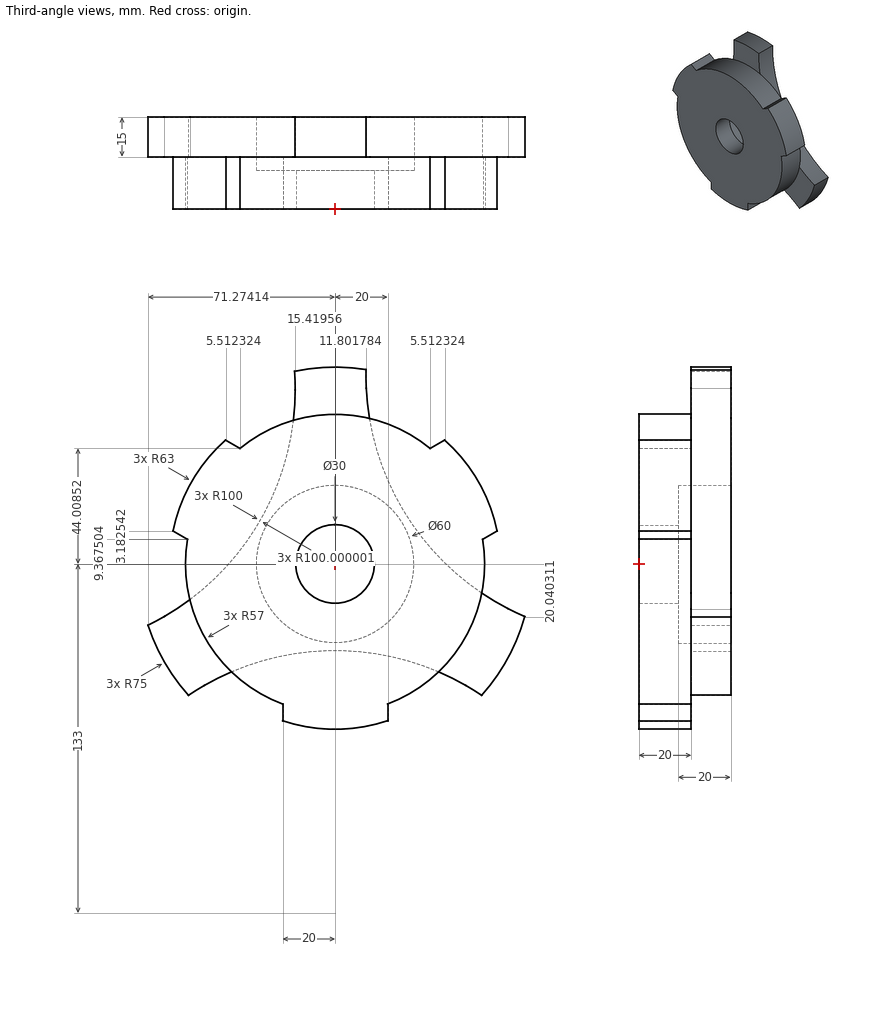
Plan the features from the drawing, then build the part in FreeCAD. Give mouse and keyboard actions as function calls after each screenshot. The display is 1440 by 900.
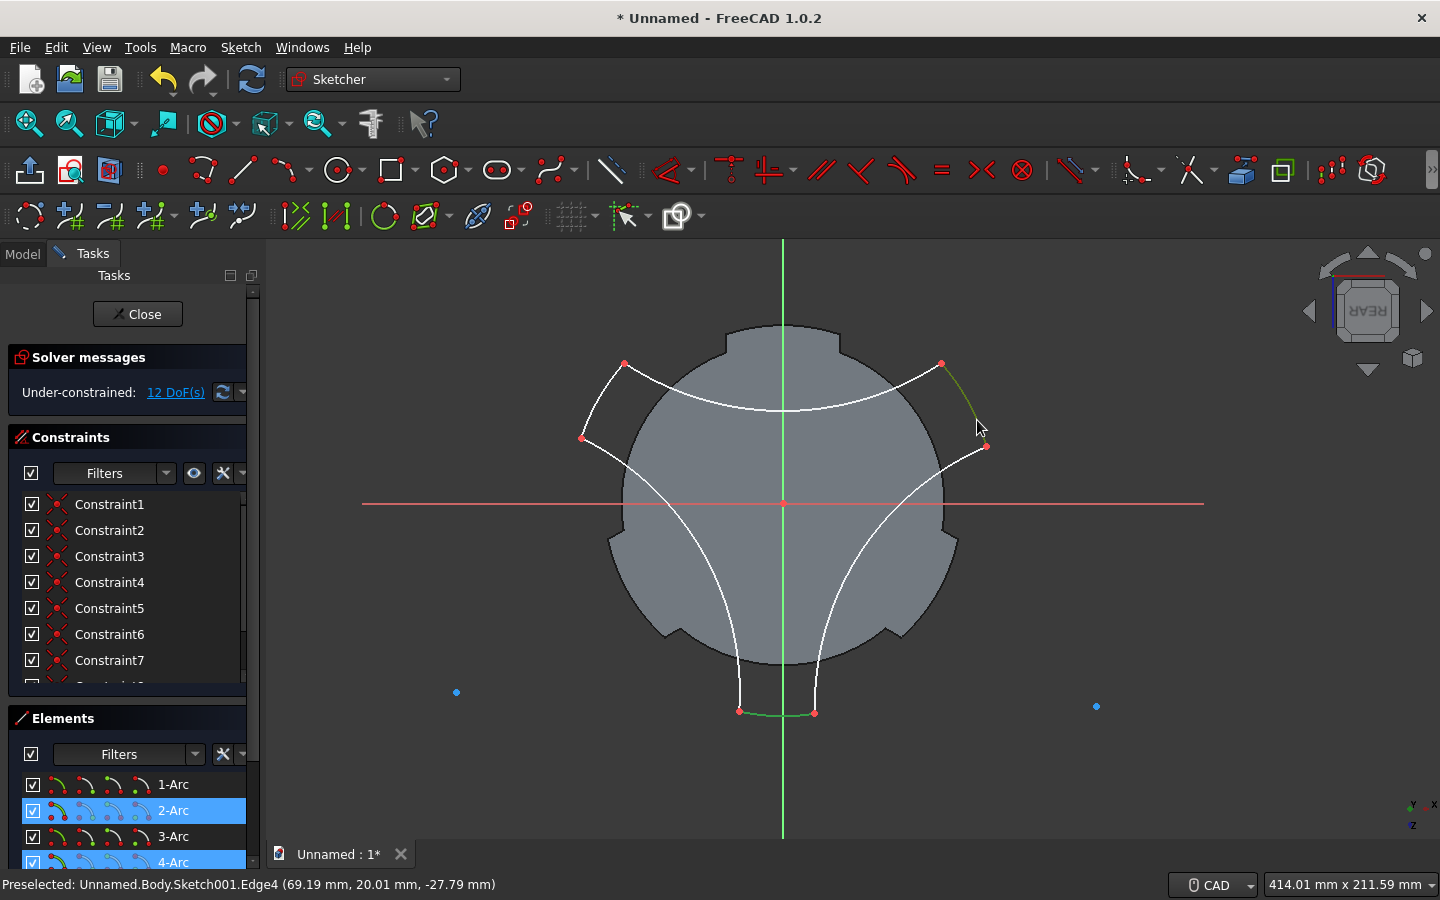
click(608, 384)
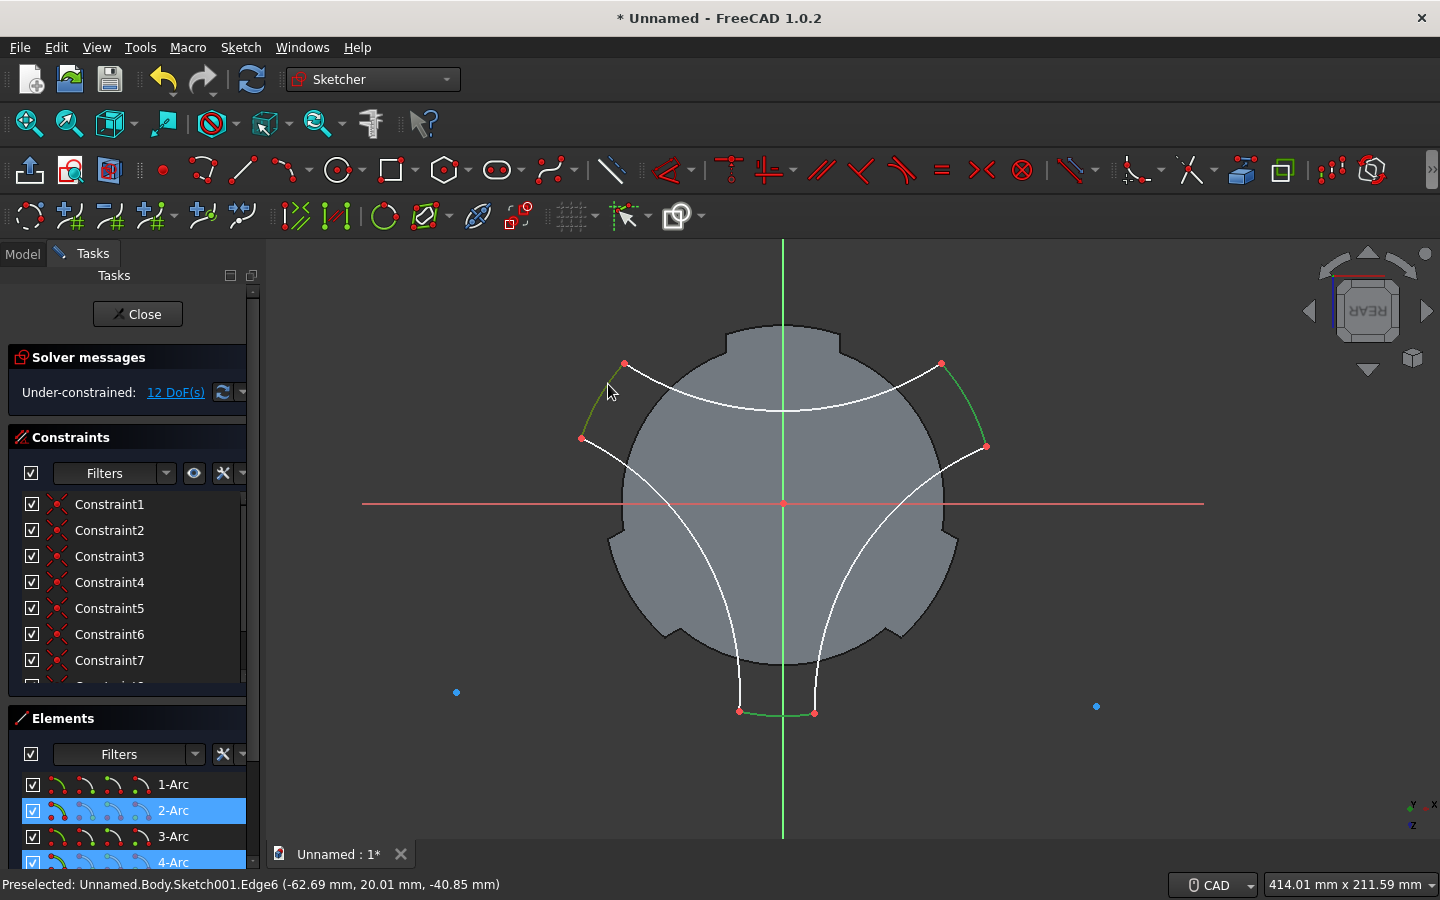
click(942, 170)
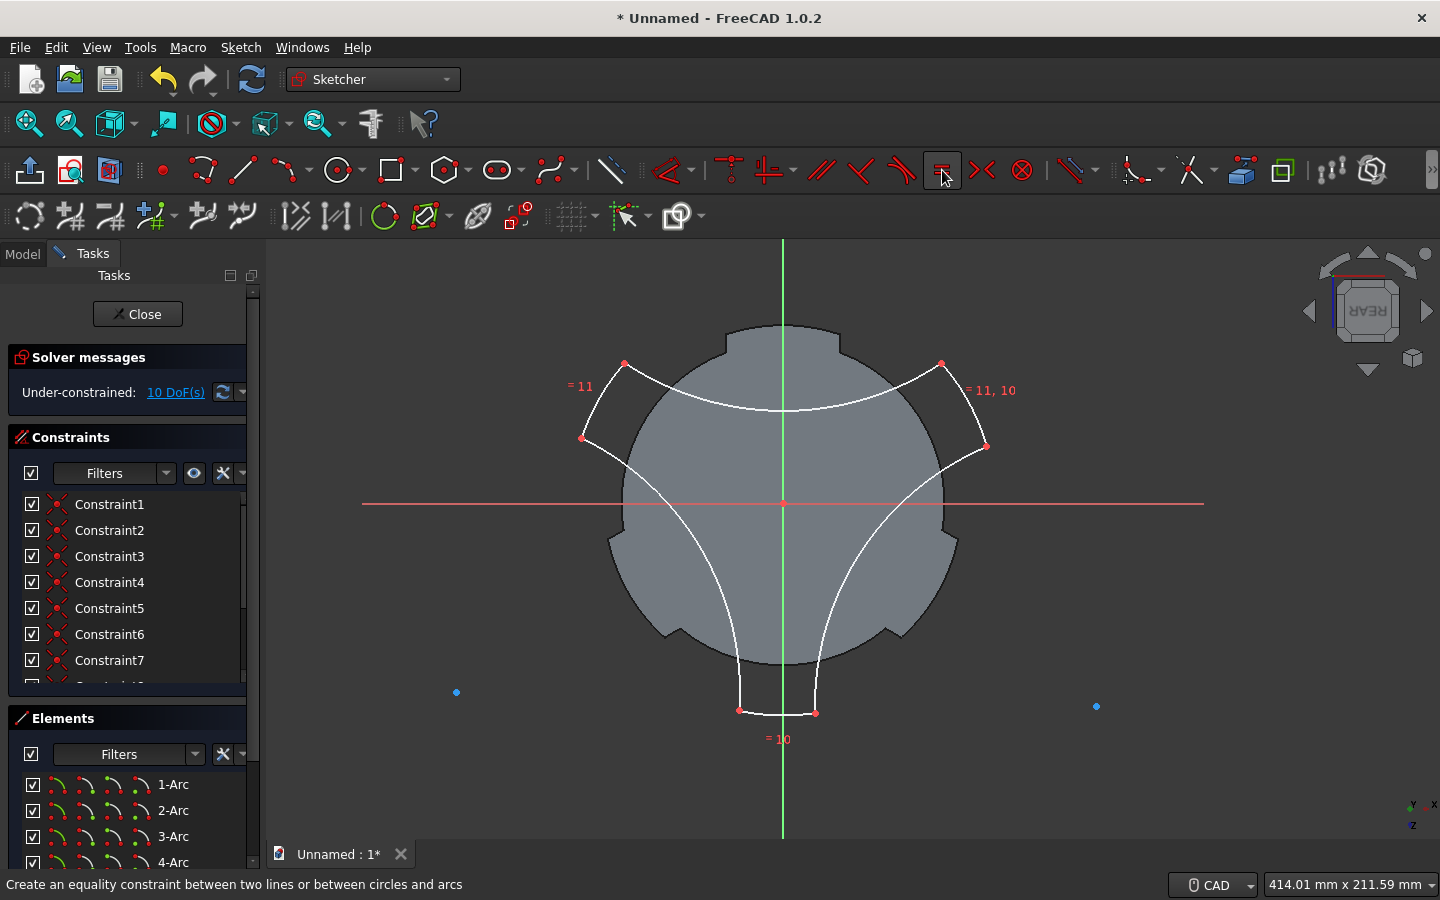
click(728, 612)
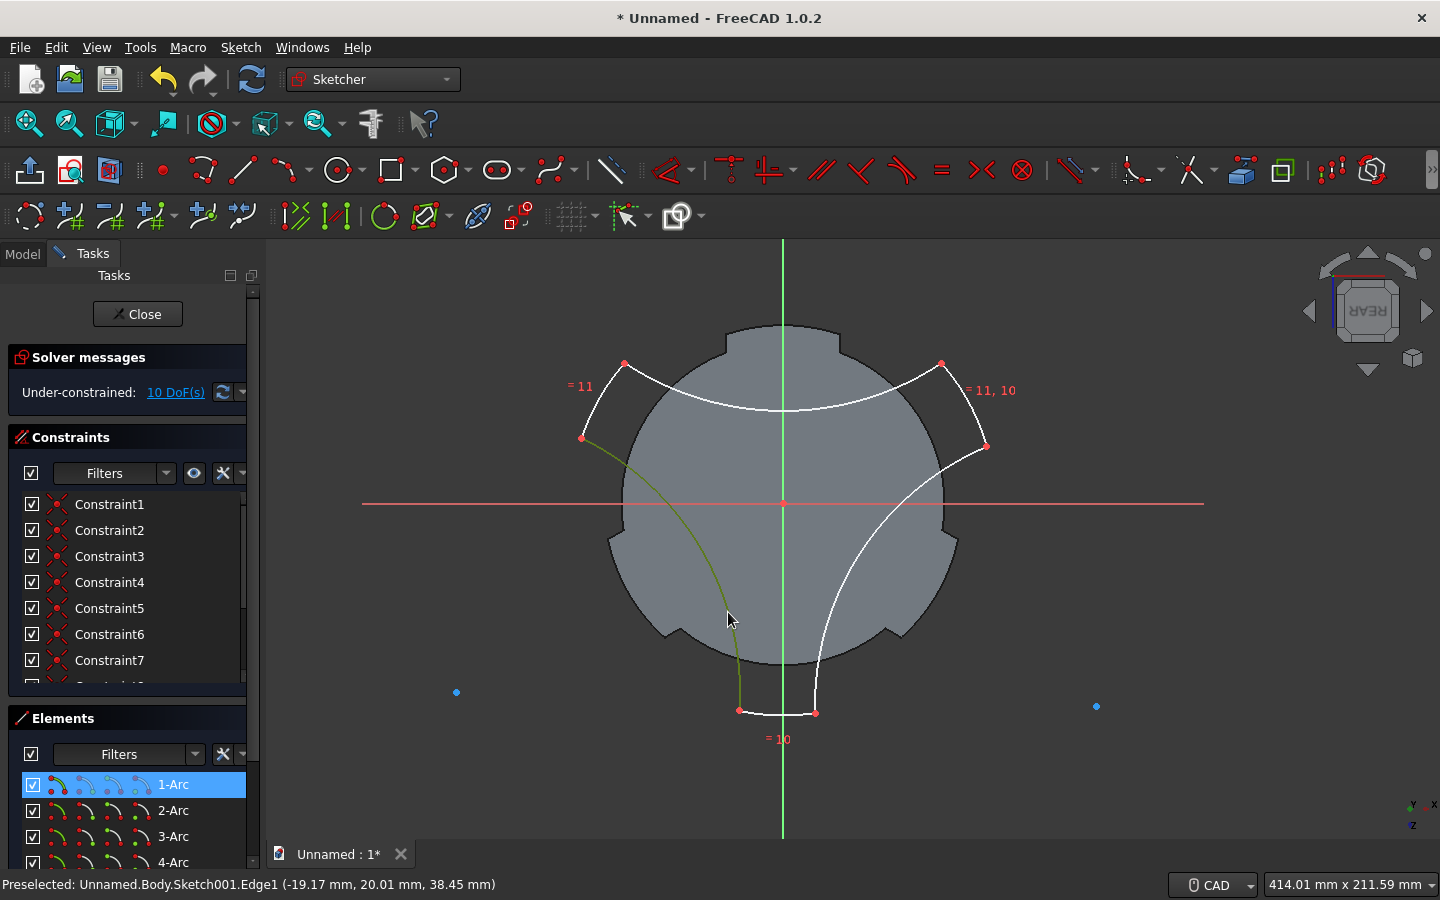
click(717, 403)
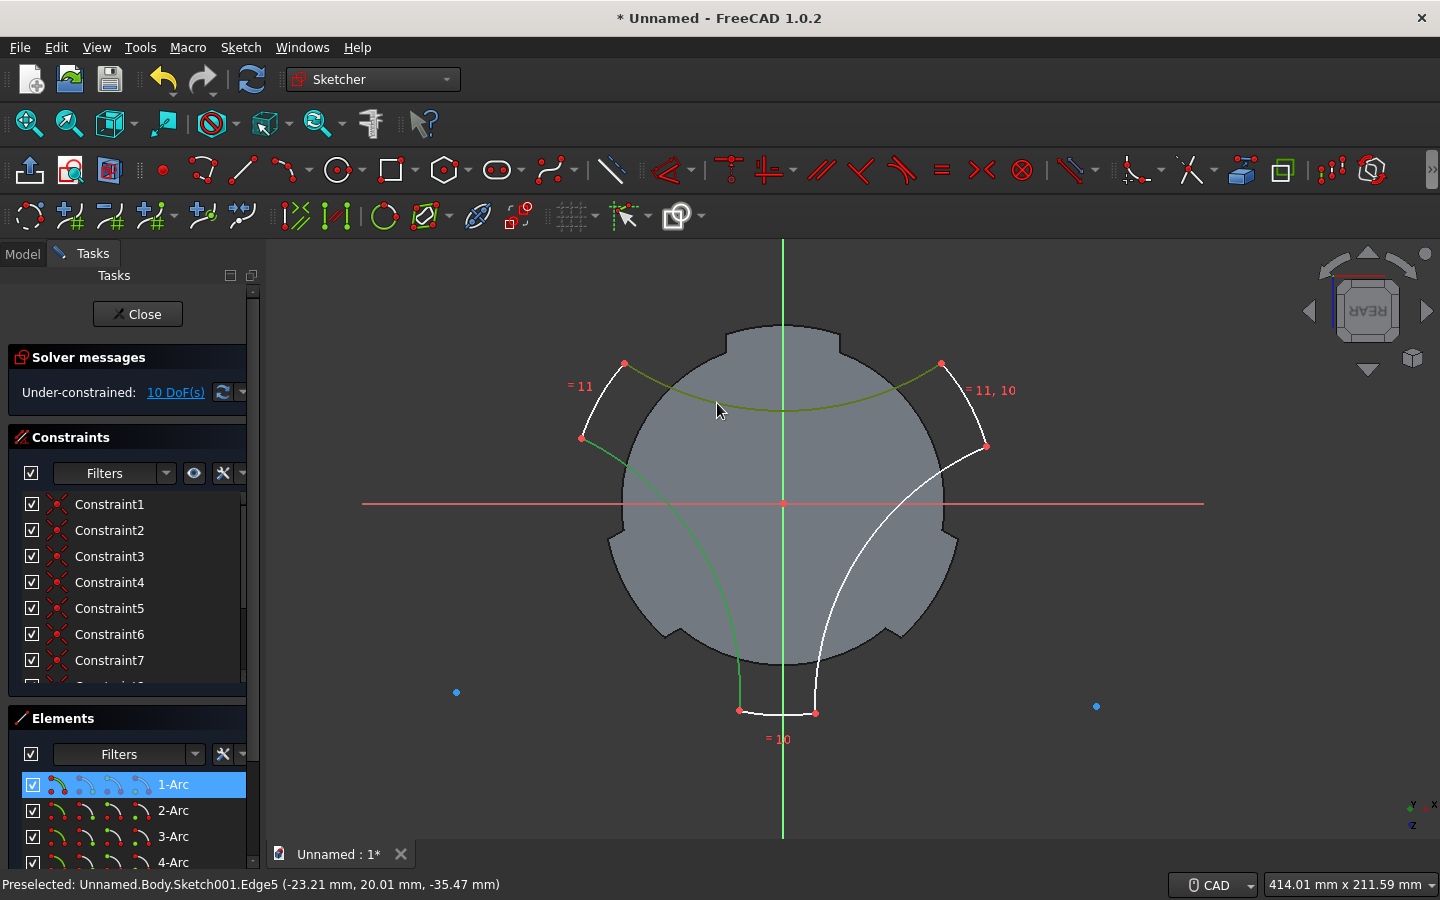
click(942, 170)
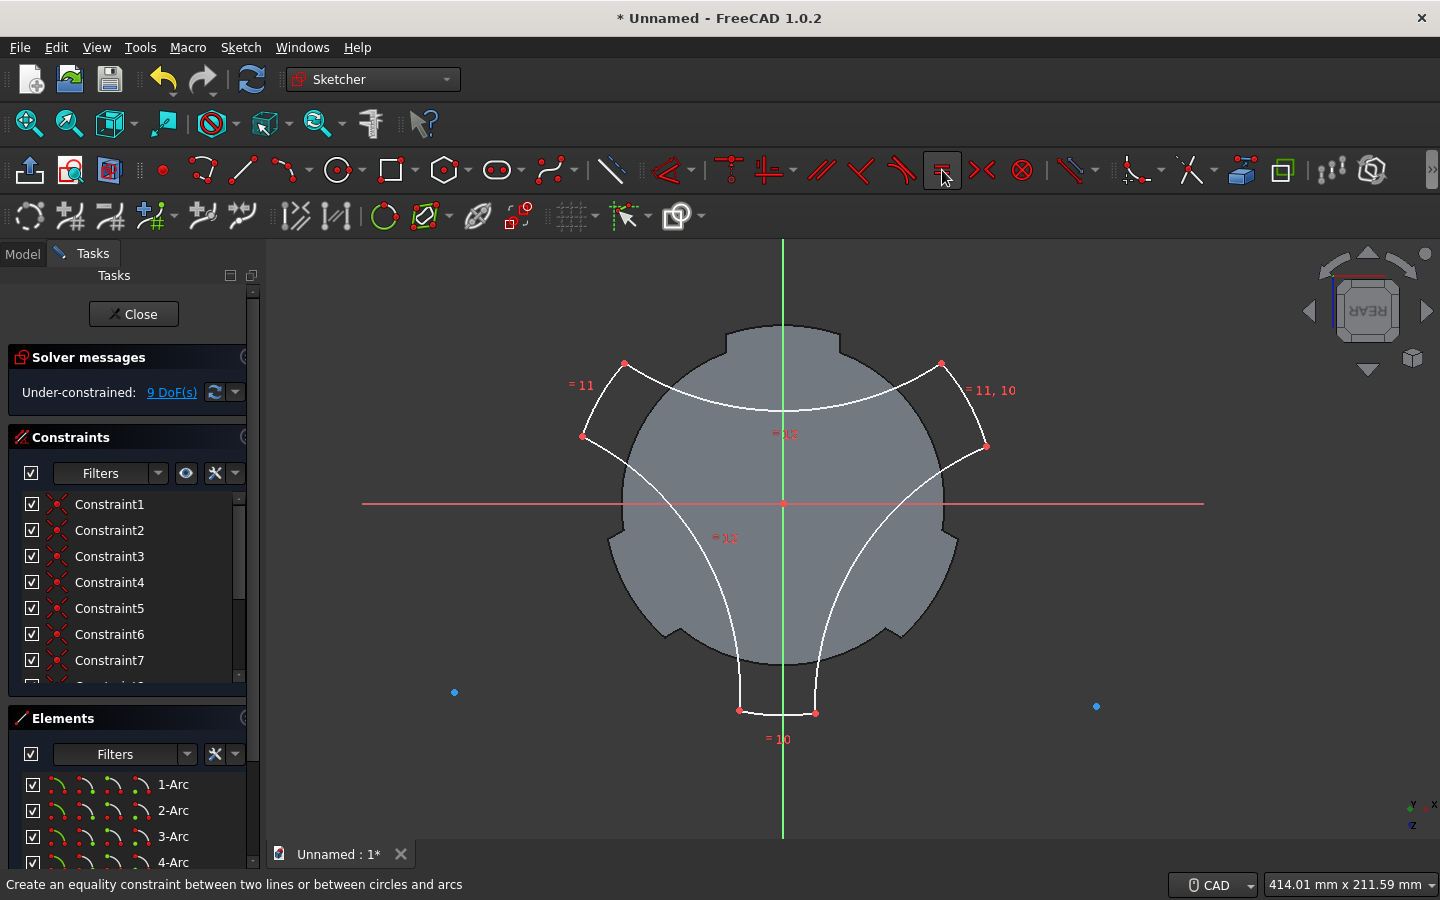
scroll(785, 780, down, 2)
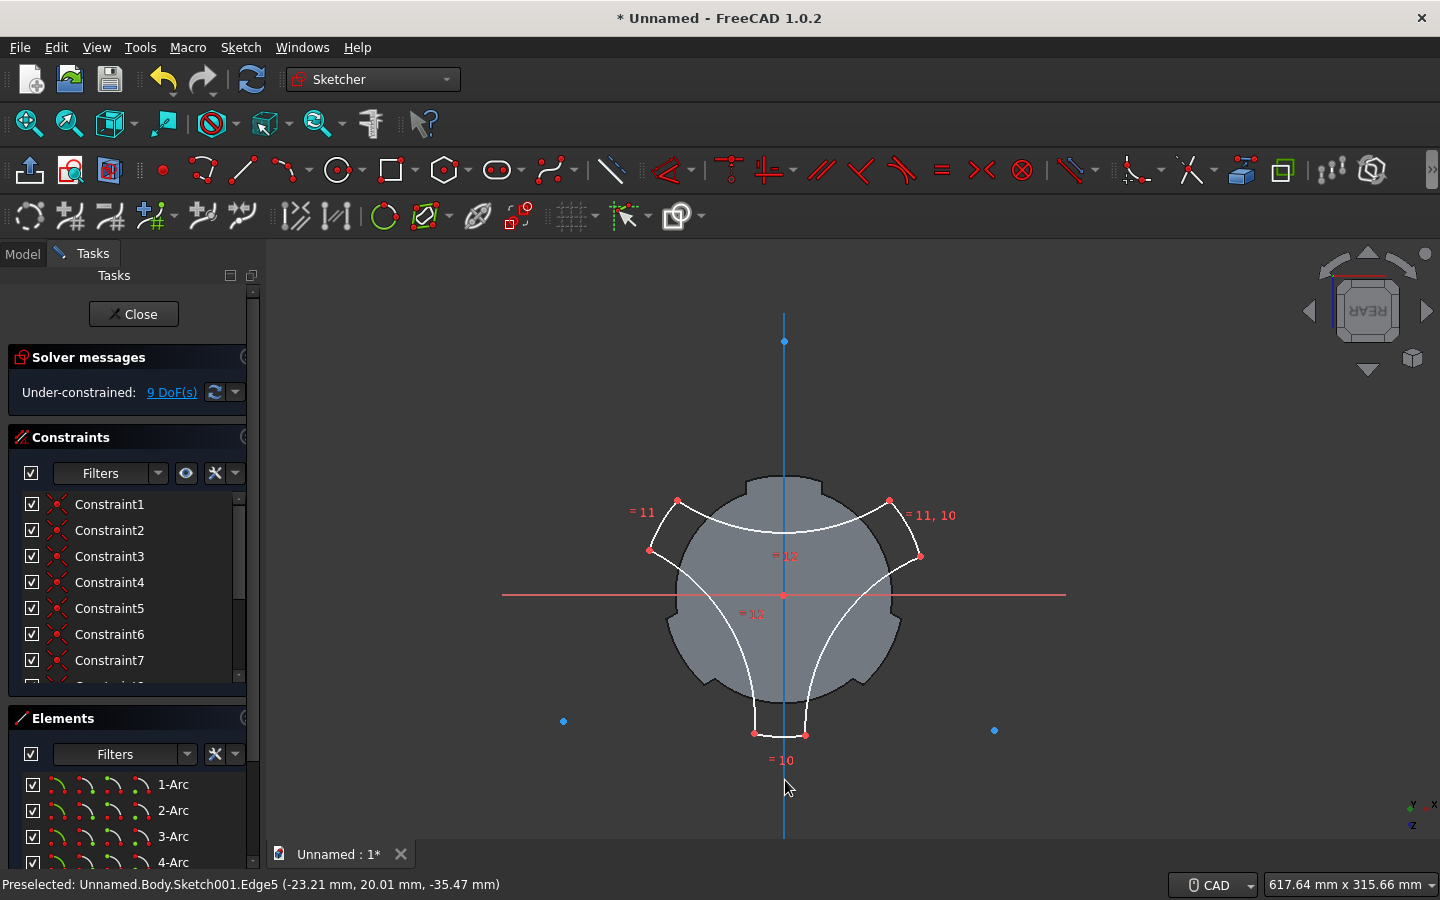
click(784, 341)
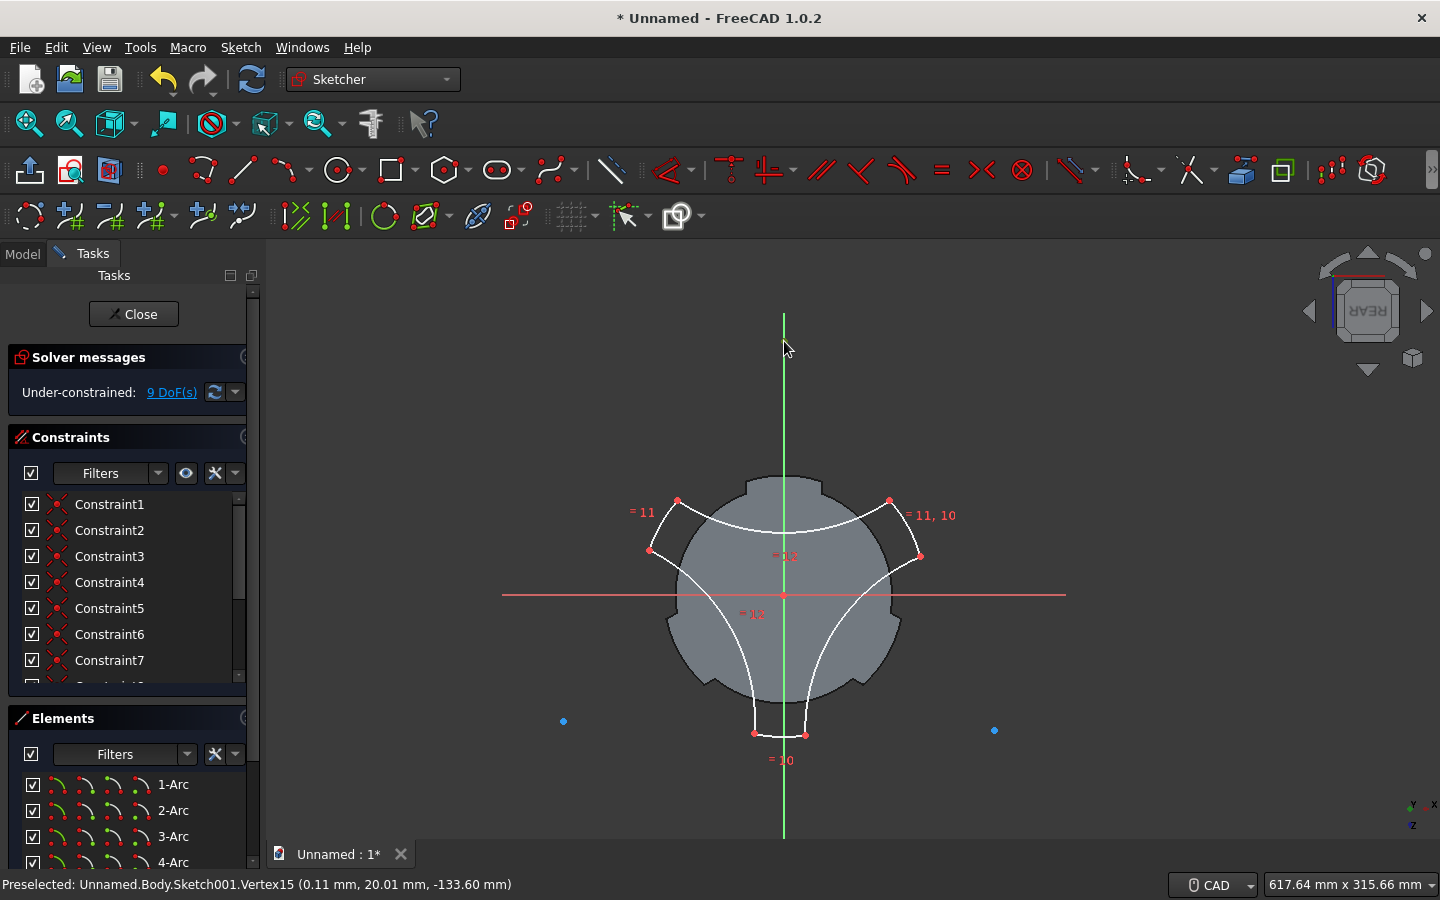
click(784, 772)